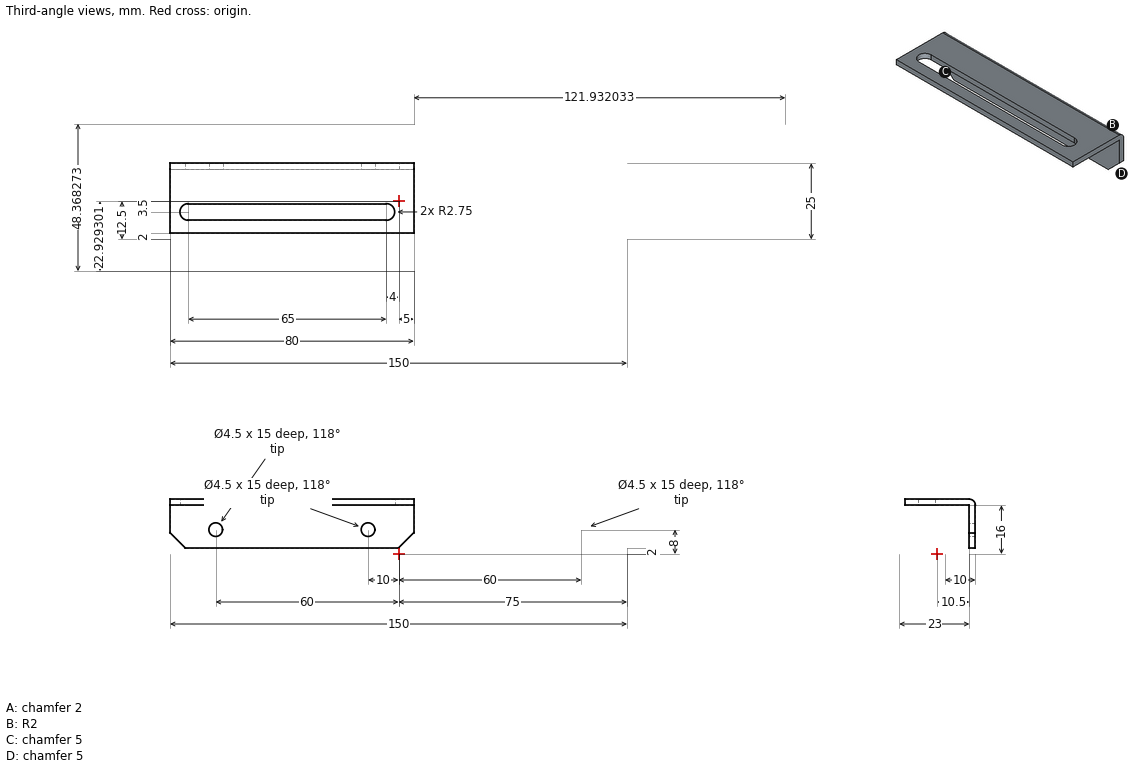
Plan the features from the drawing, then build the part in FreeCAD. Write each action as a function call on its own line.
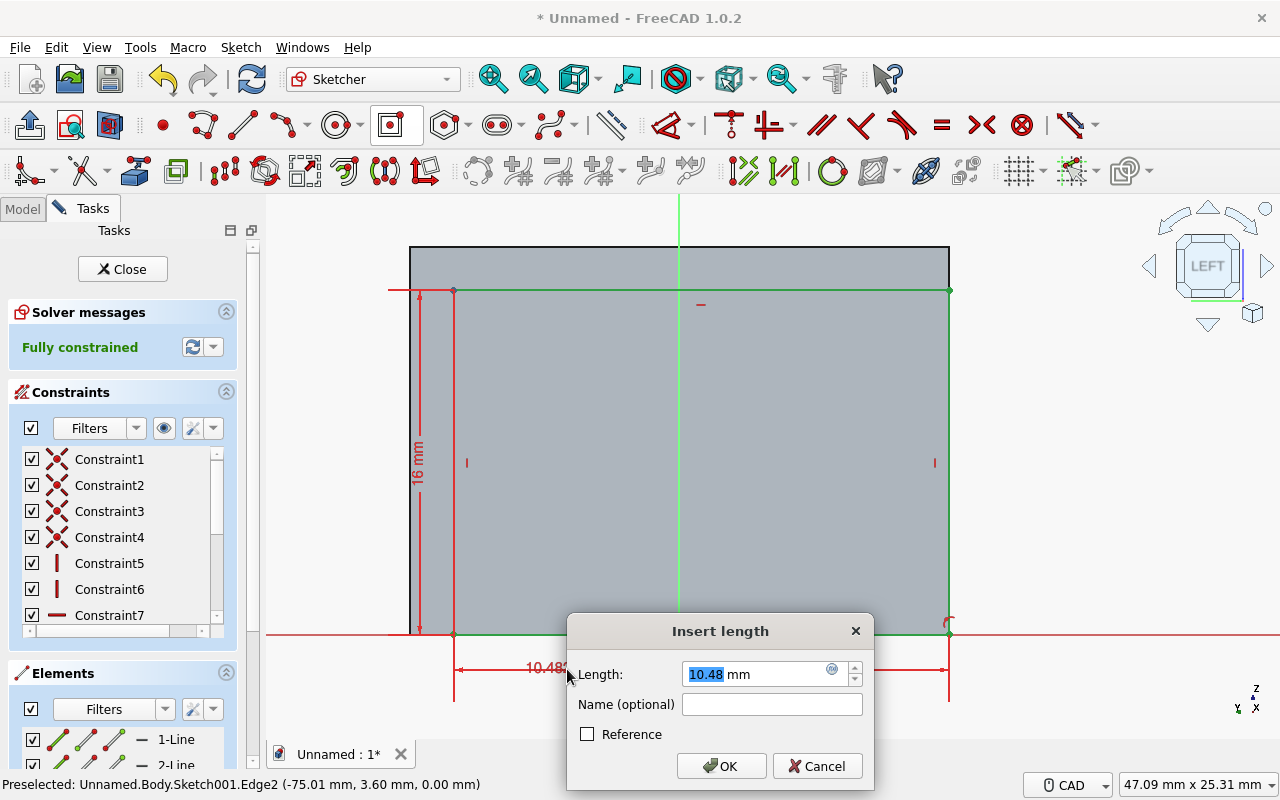
text(10.5)
key(Return)
key(Escape)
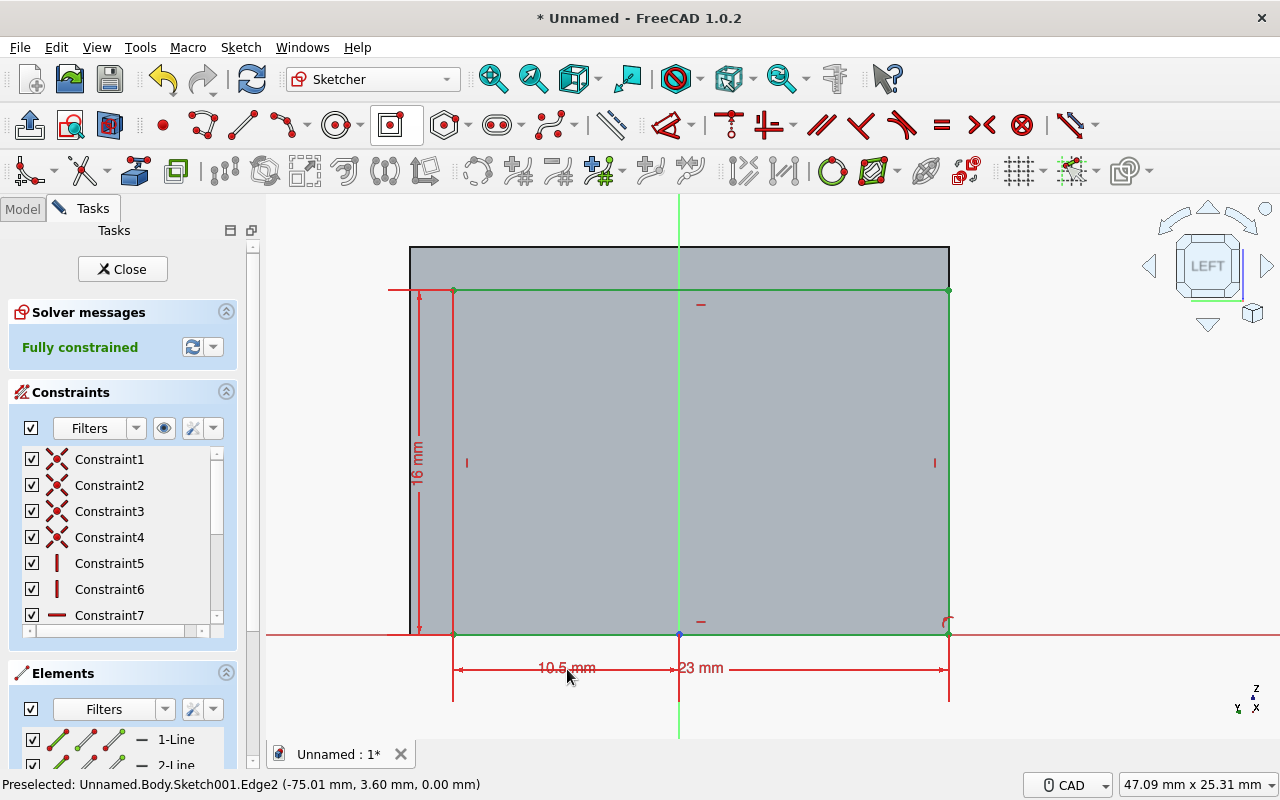
click(123, 269)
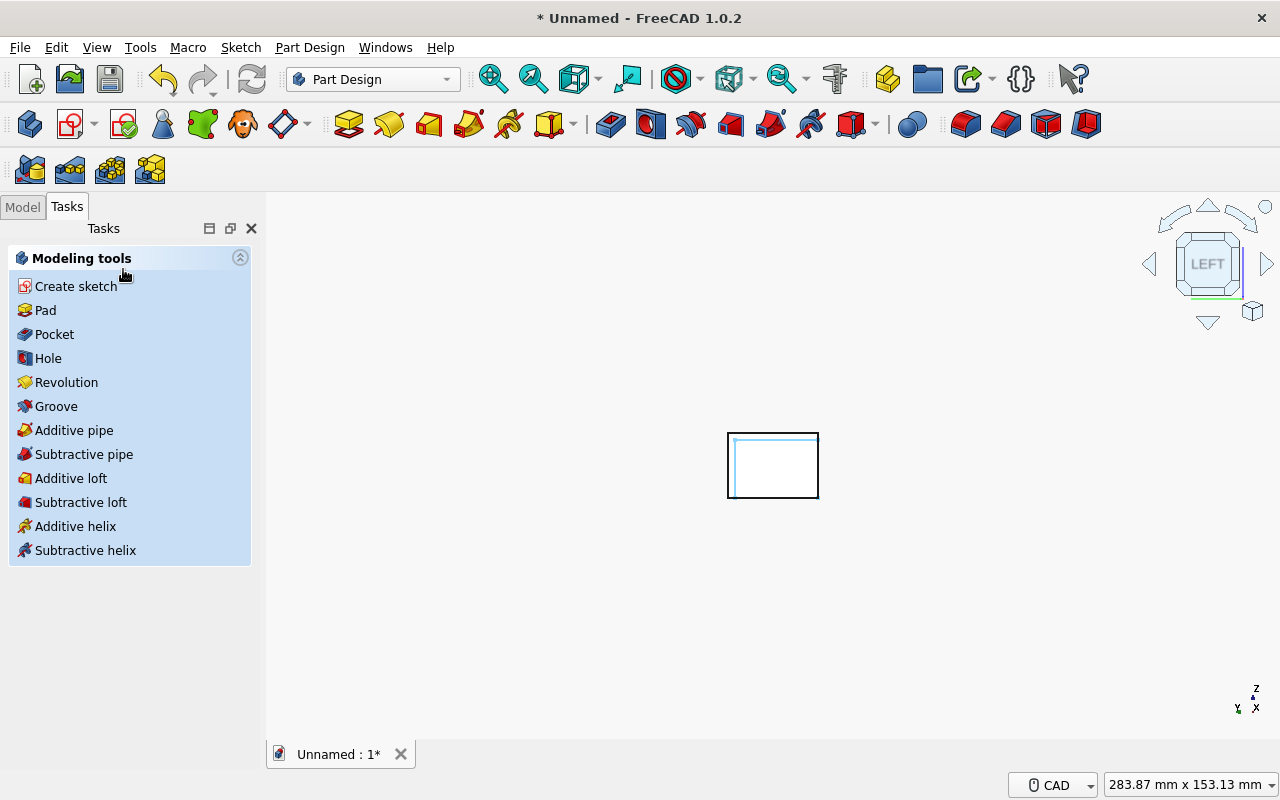
click(612, 124)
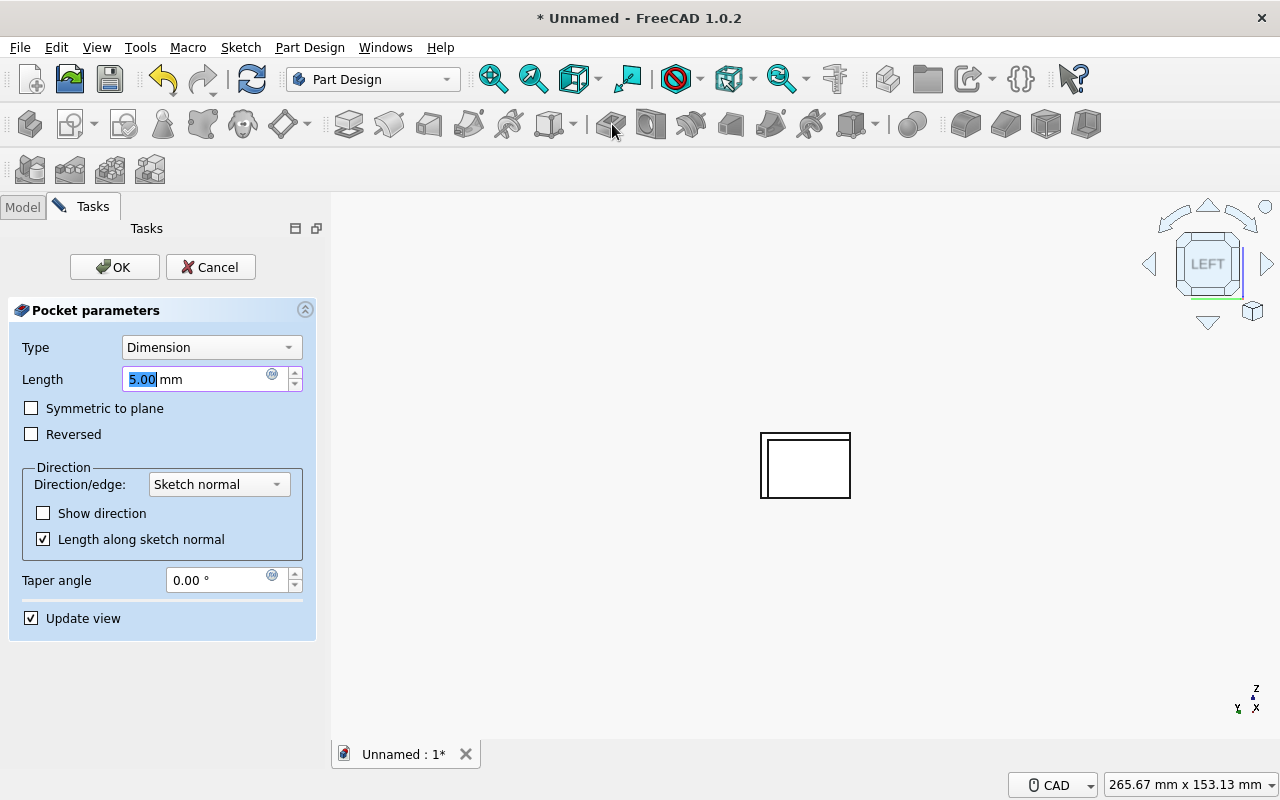
click(212, 348)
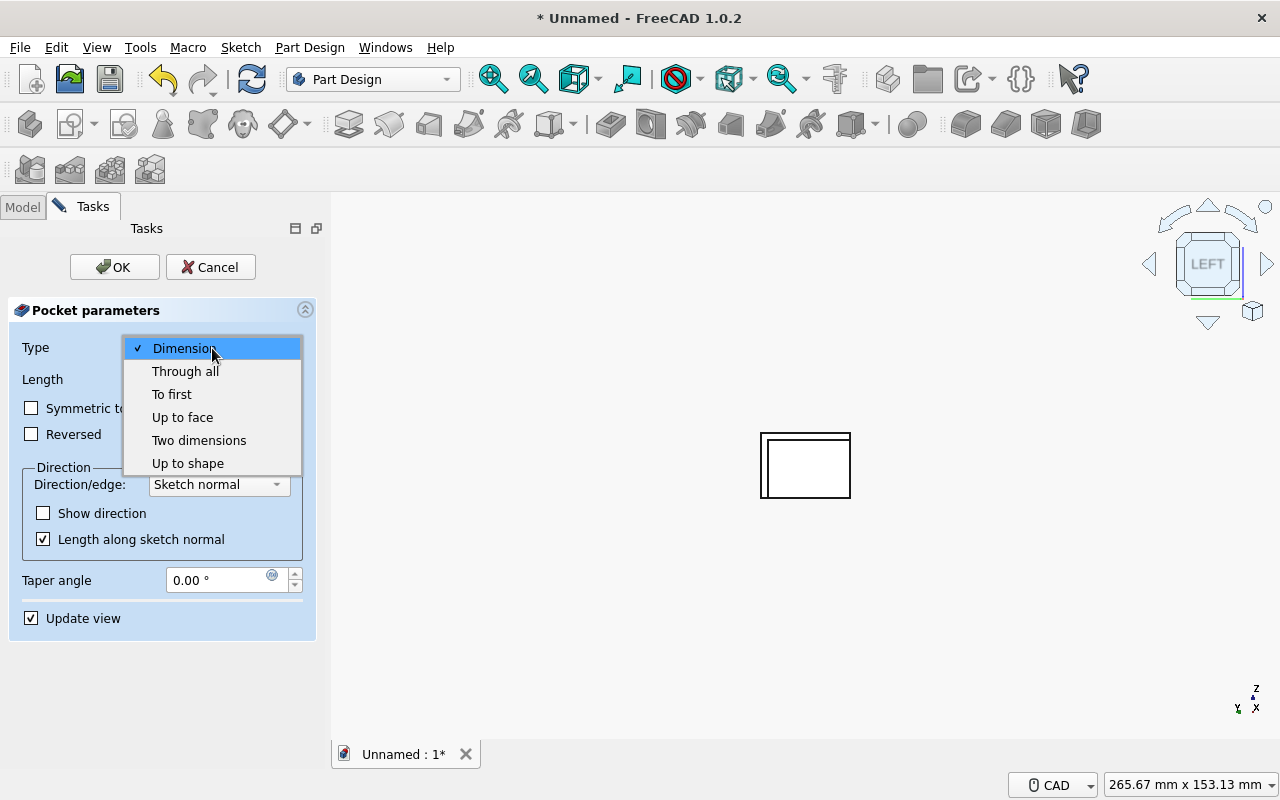
click(212, 372)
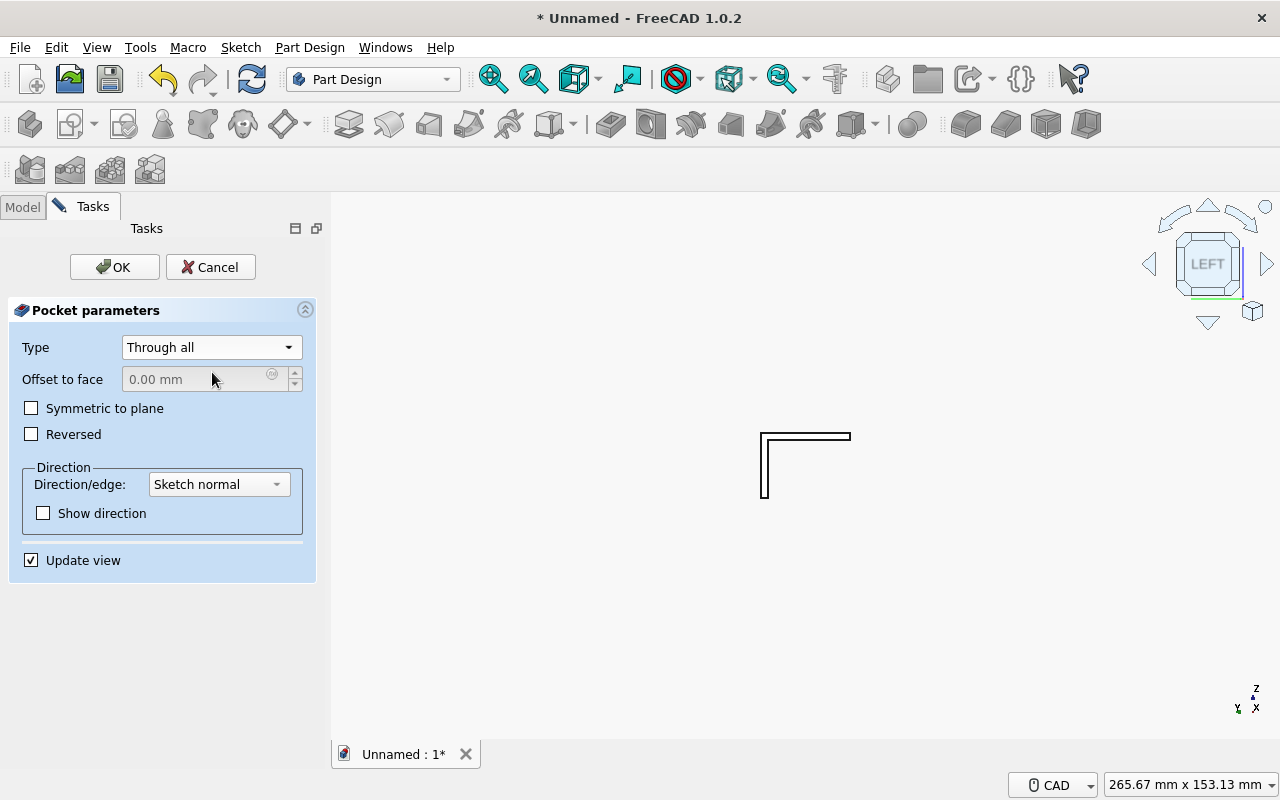
click(115, 267)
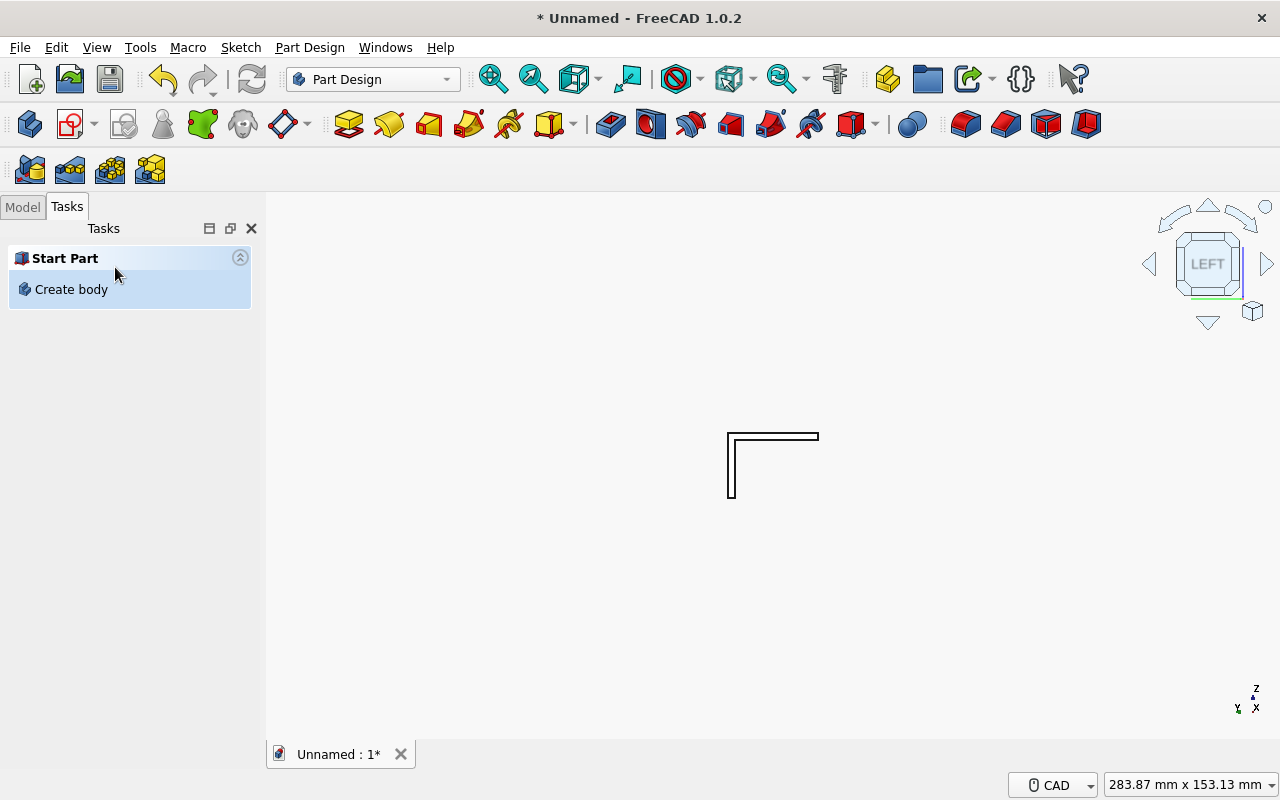
key(v)
key(f)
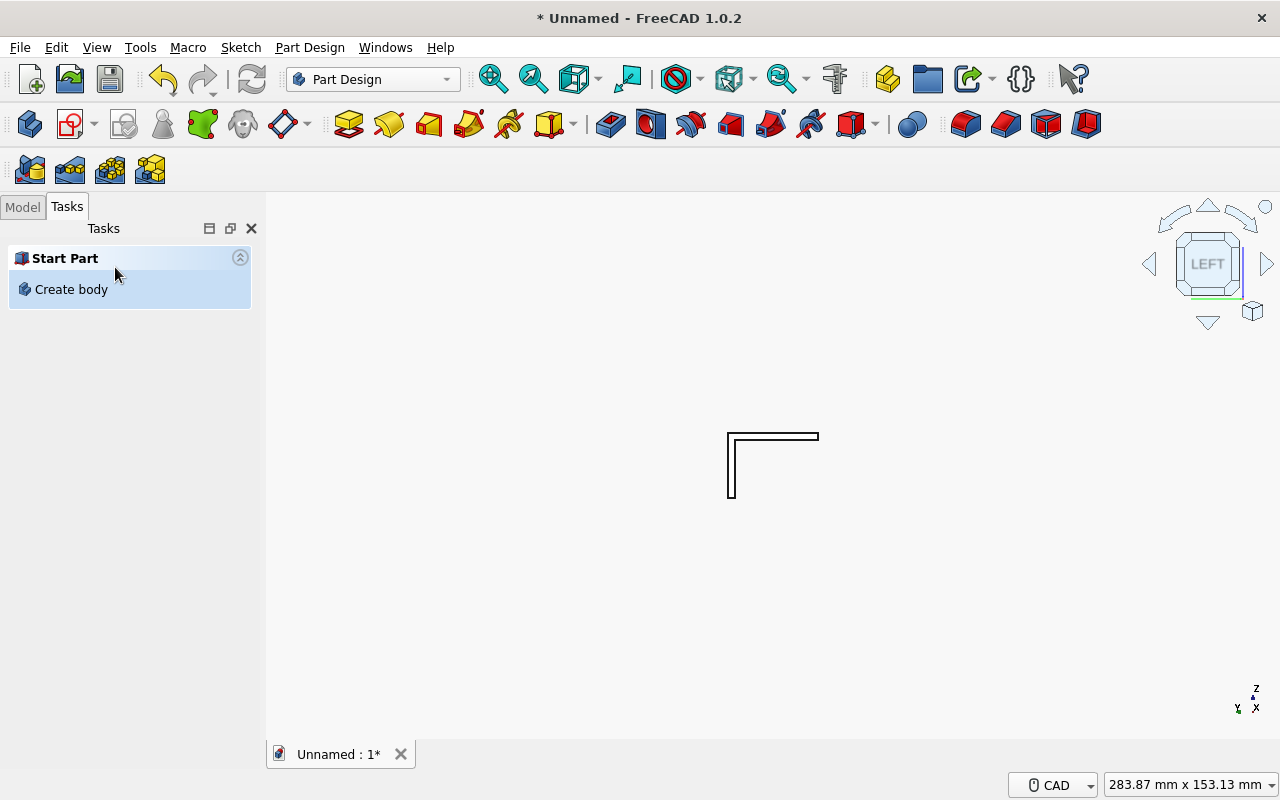
key(0)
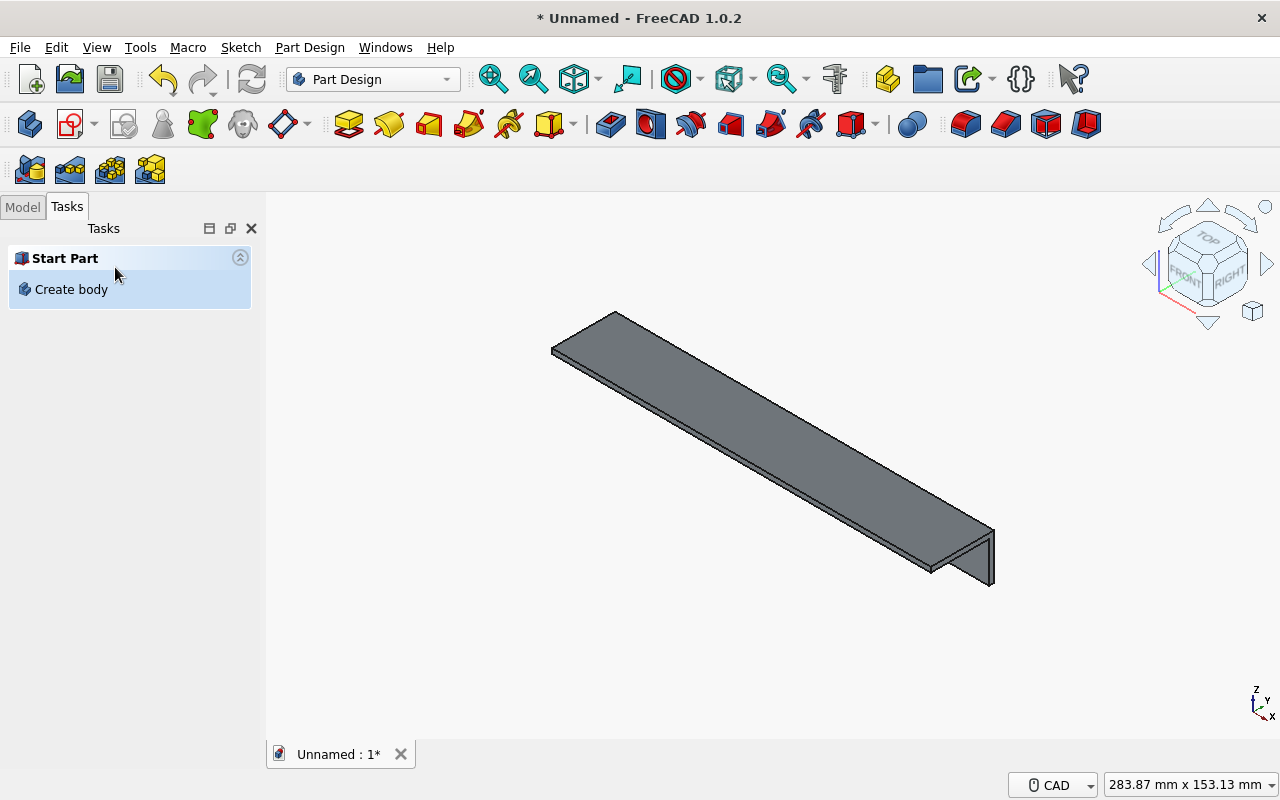
click(881, 501)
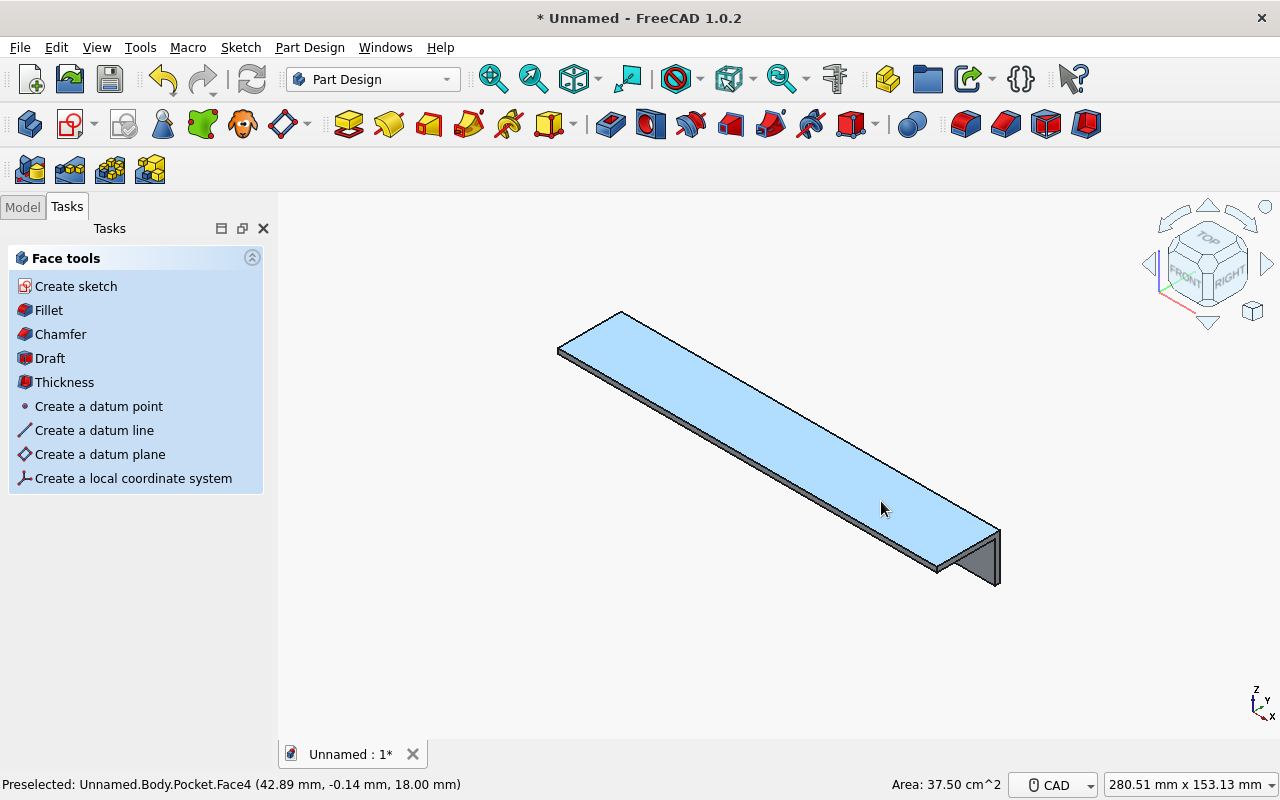
click(70, 124)